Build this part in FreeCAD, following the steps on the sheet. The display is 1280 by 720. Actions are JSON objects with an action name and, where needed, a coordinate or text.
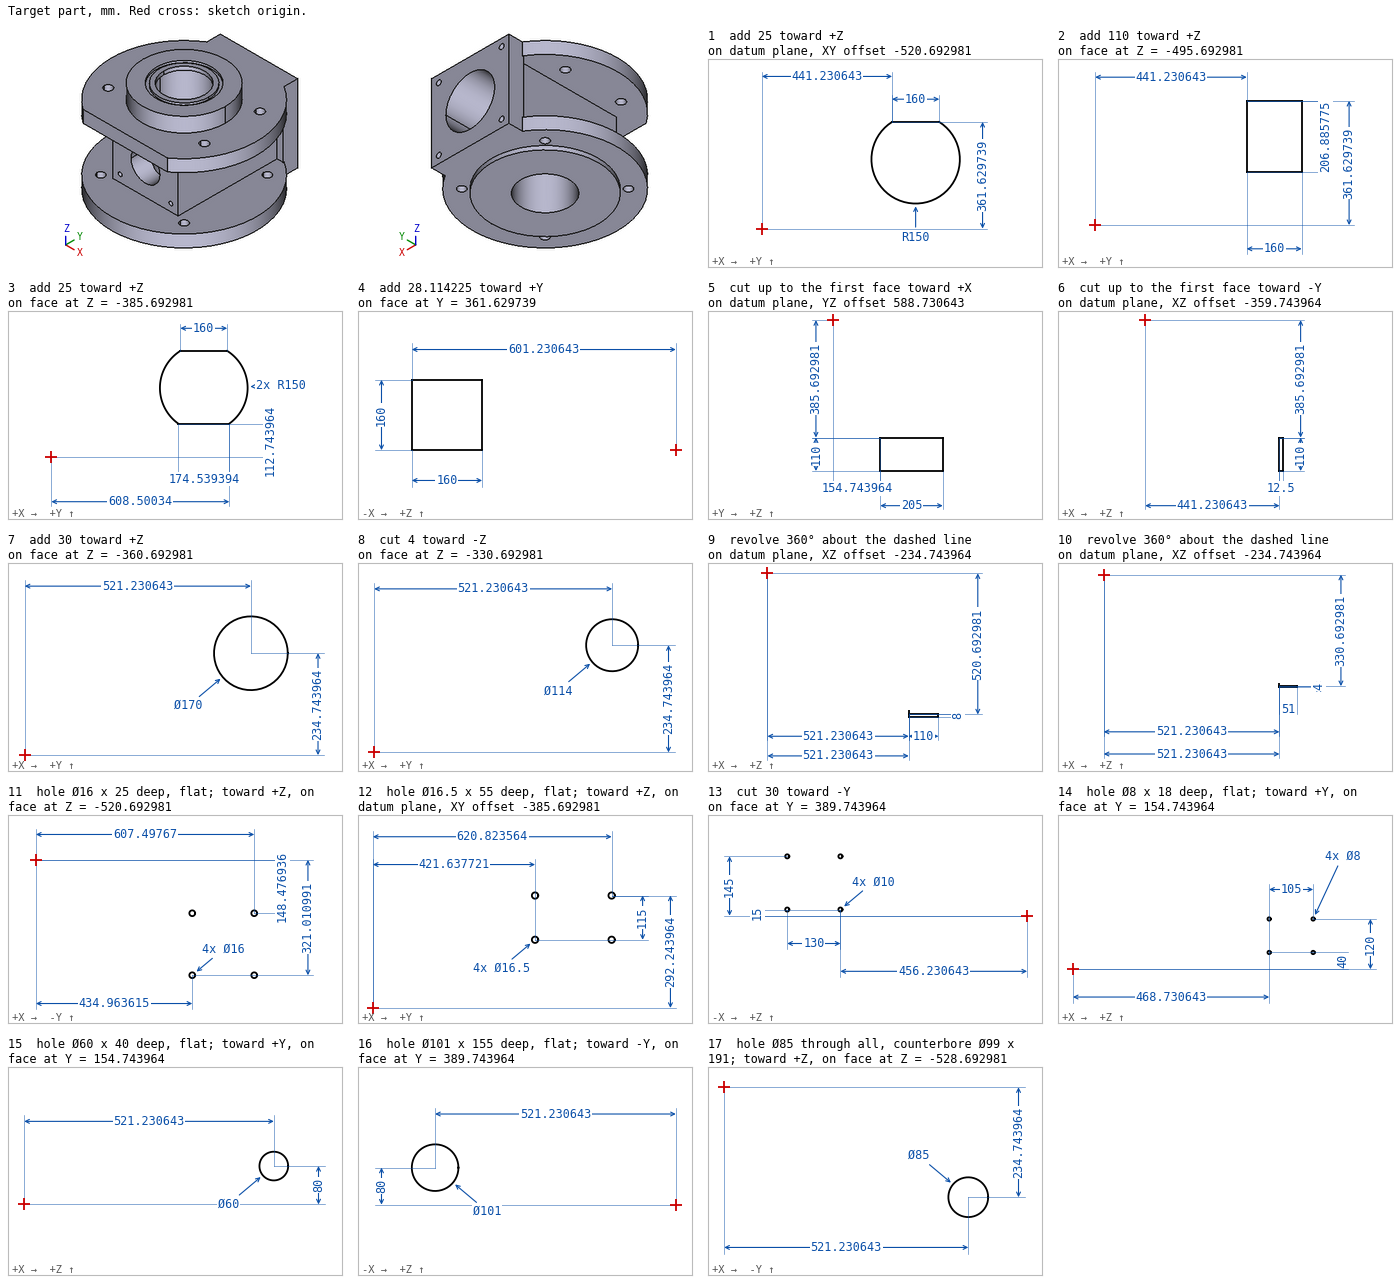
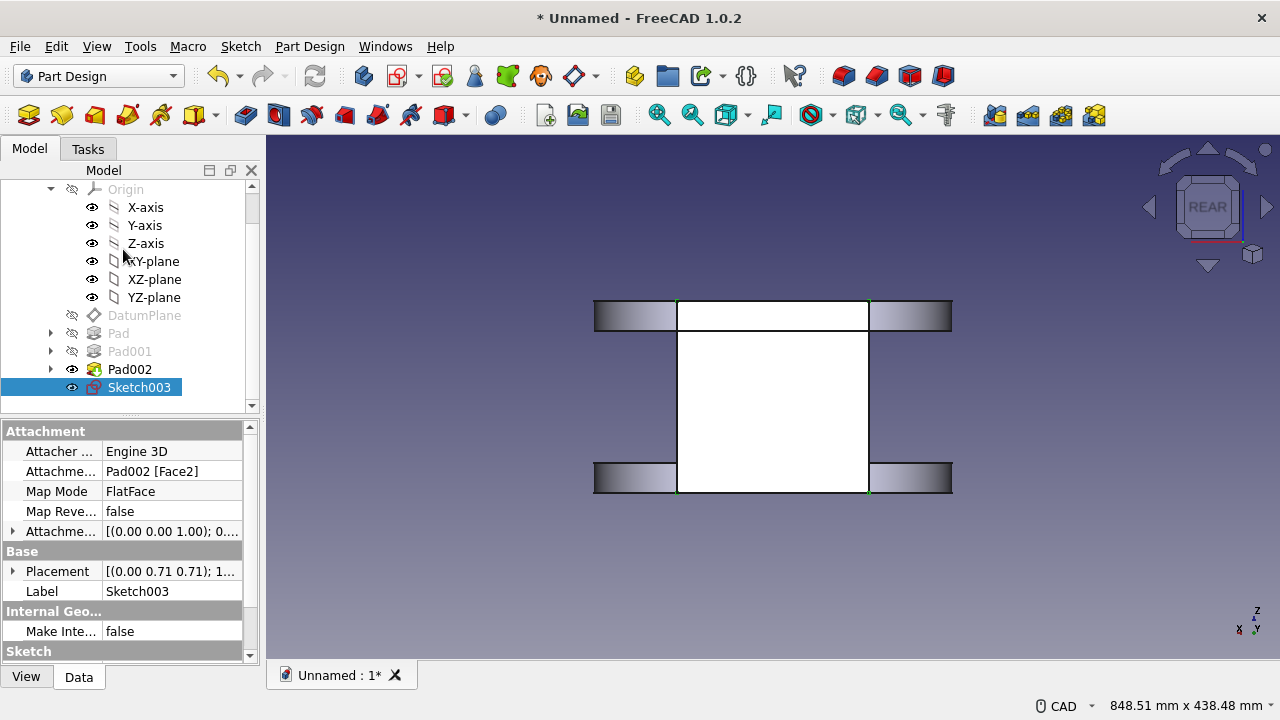
{"action": "left_click", "coordinate": [29, 116]}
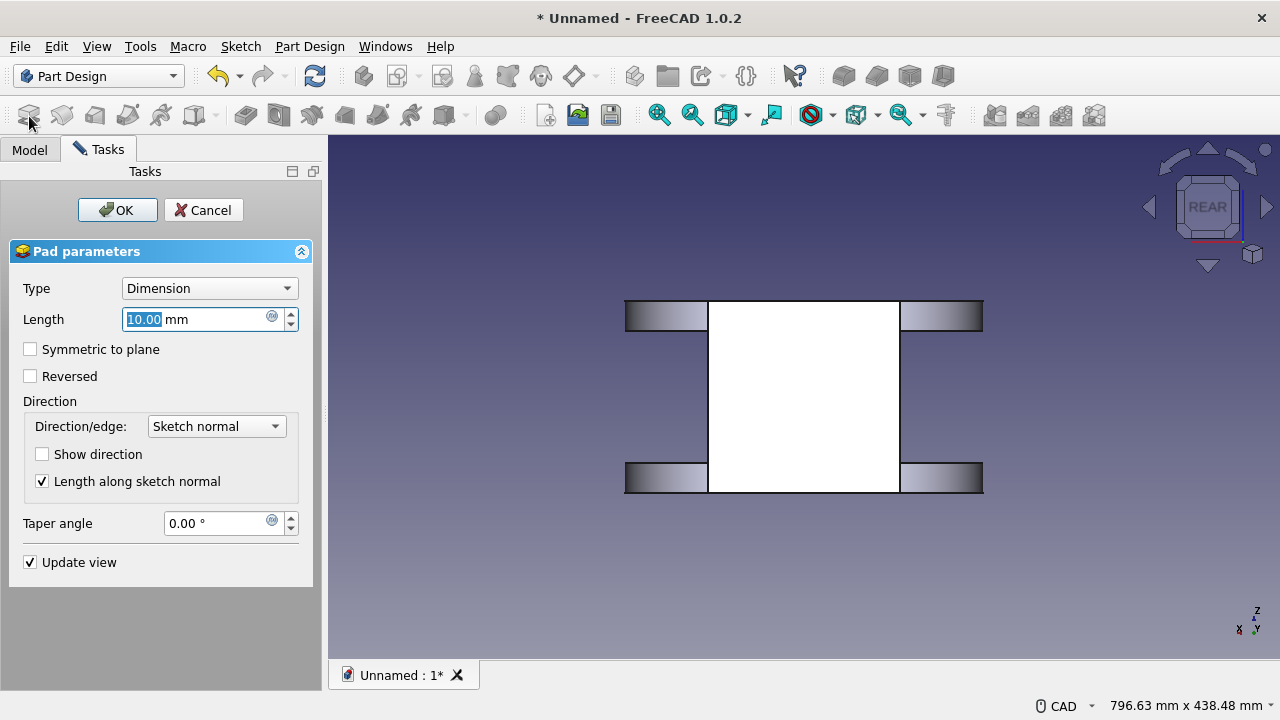
{"action": "type", "text": "28.114225"}
{"action": "key", "text": "Tab"}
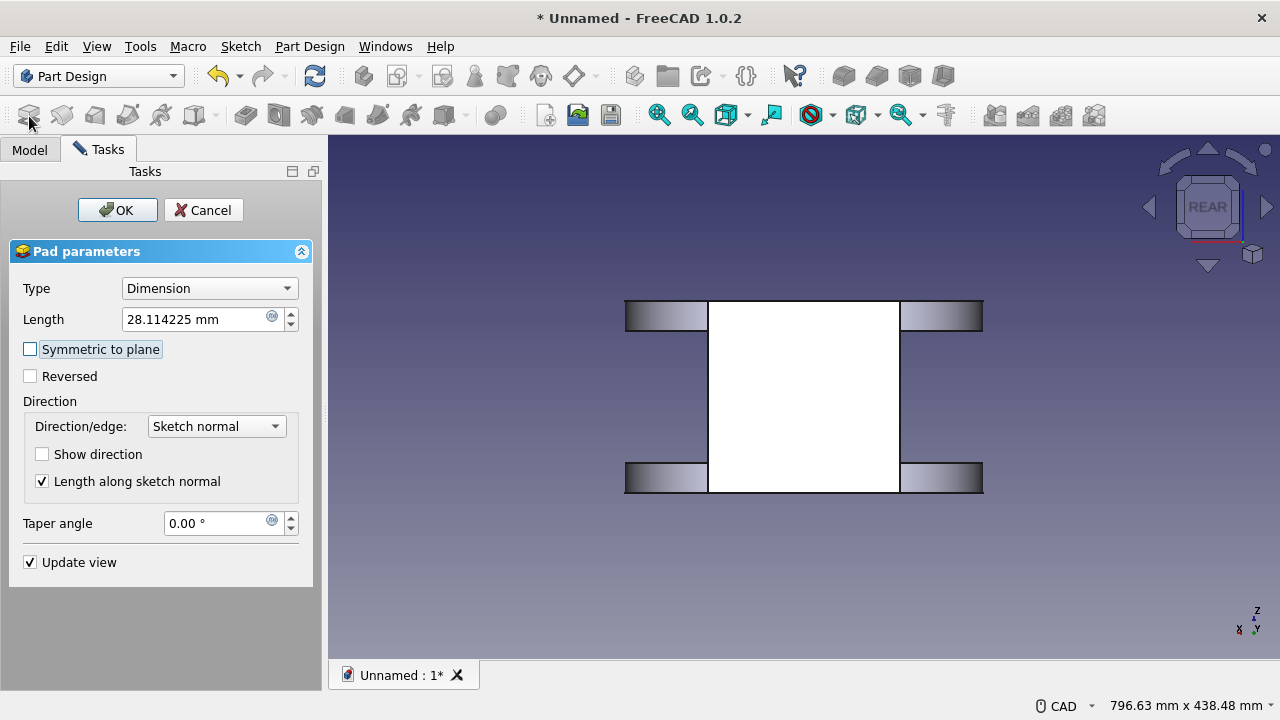
{"action": "left_click", "coordinate": [118, 210]}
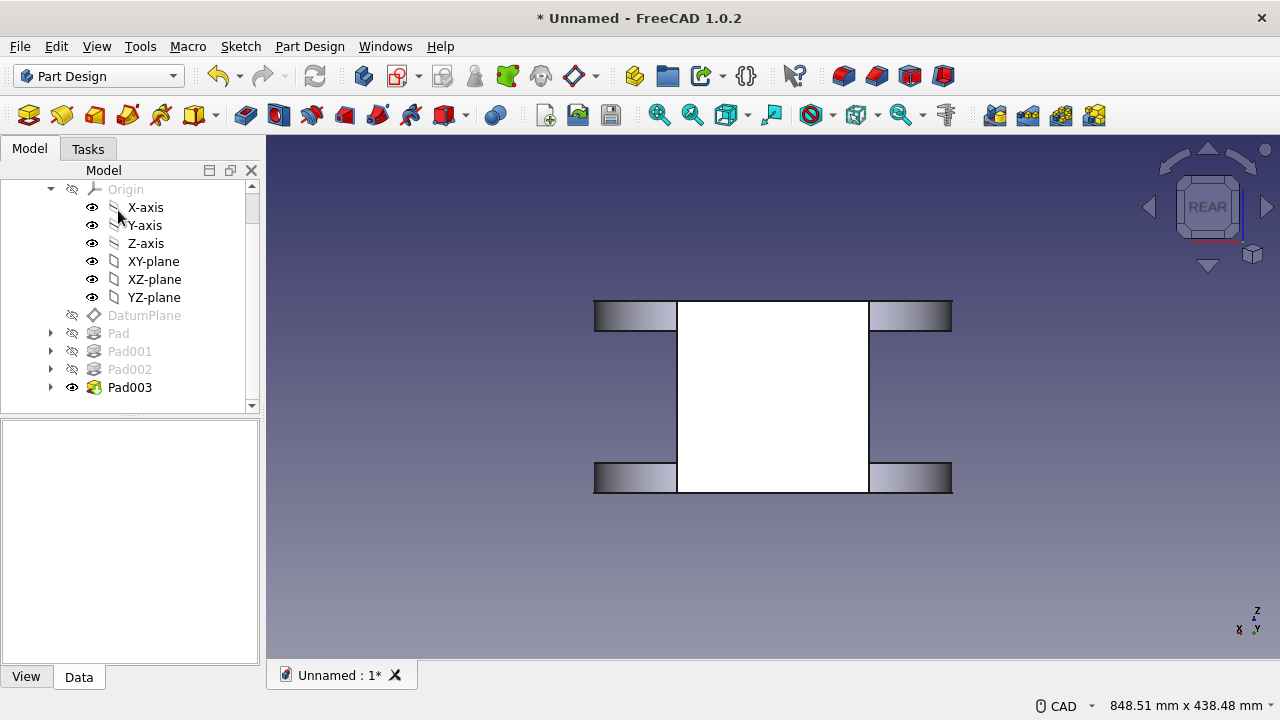
{"action": "left_click", "coordinate": [660, 116]}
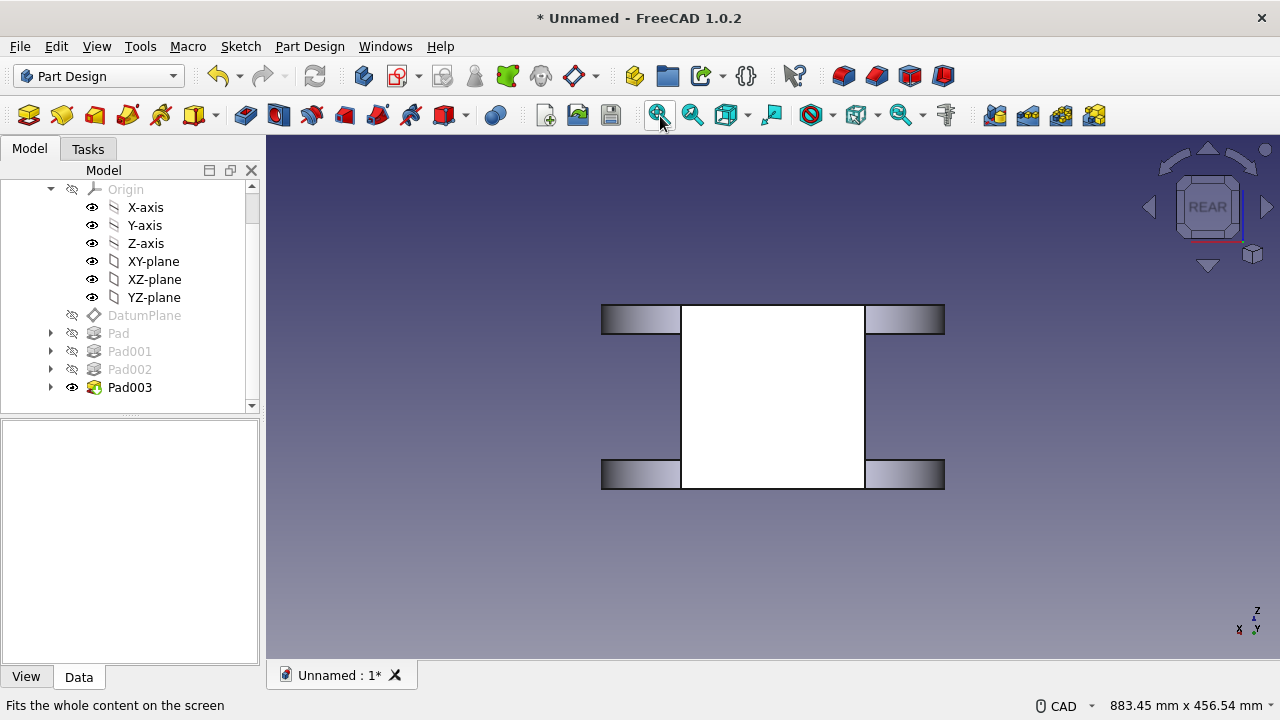
{"action": "left_click", "coordinate": [137, 297]}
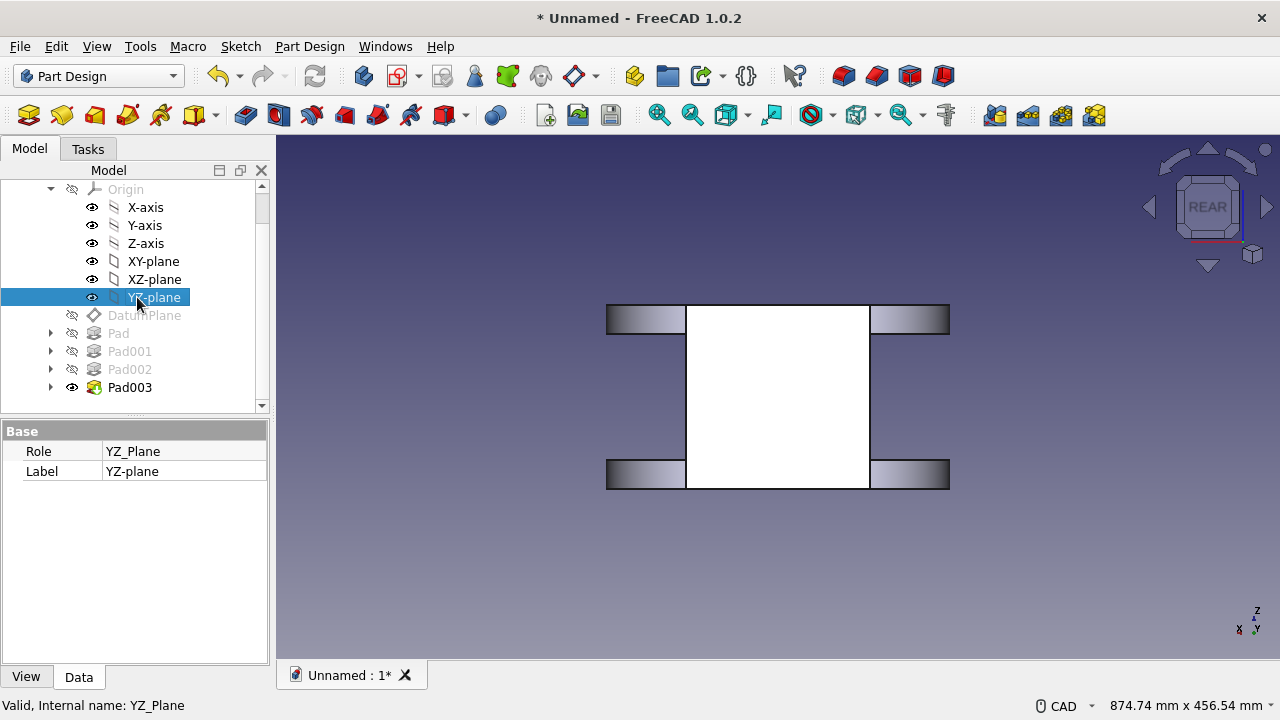
{"action": "left_click", "coordinate": [574, 76]}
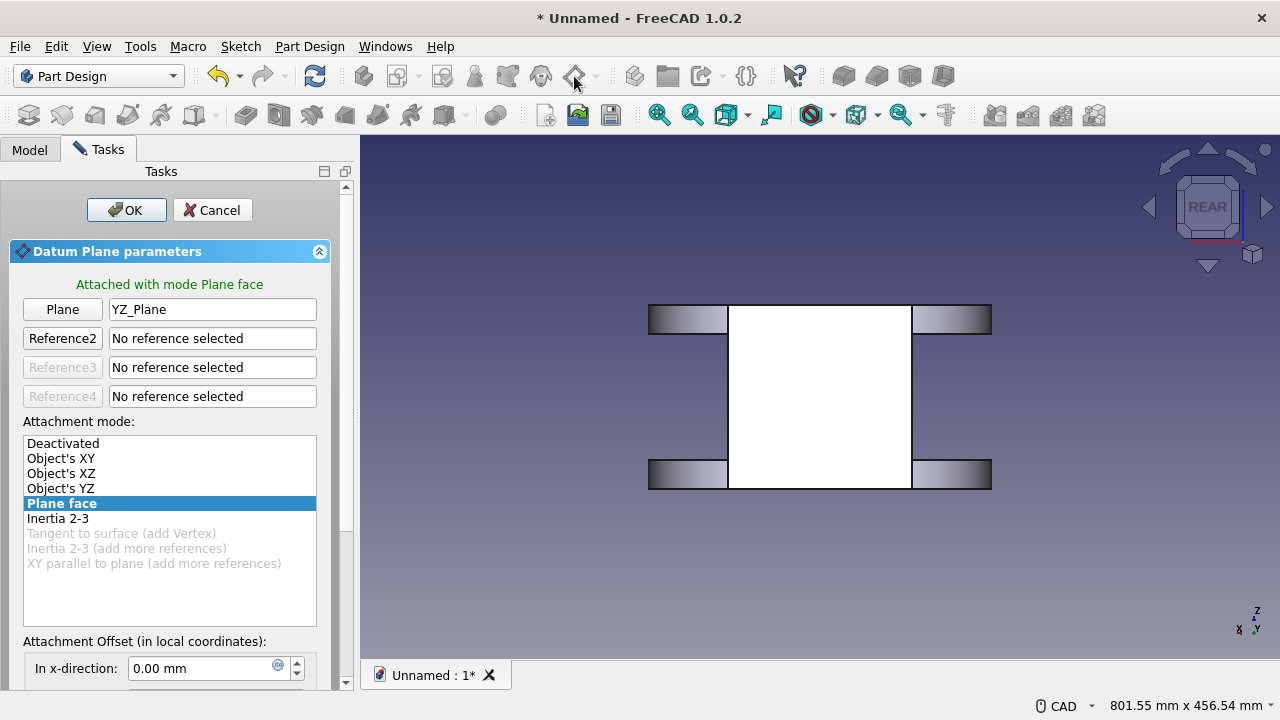
{"action": "scroll", "coordinate": [346, 436], "scroll_direction": "down", "scroll_amount": 2}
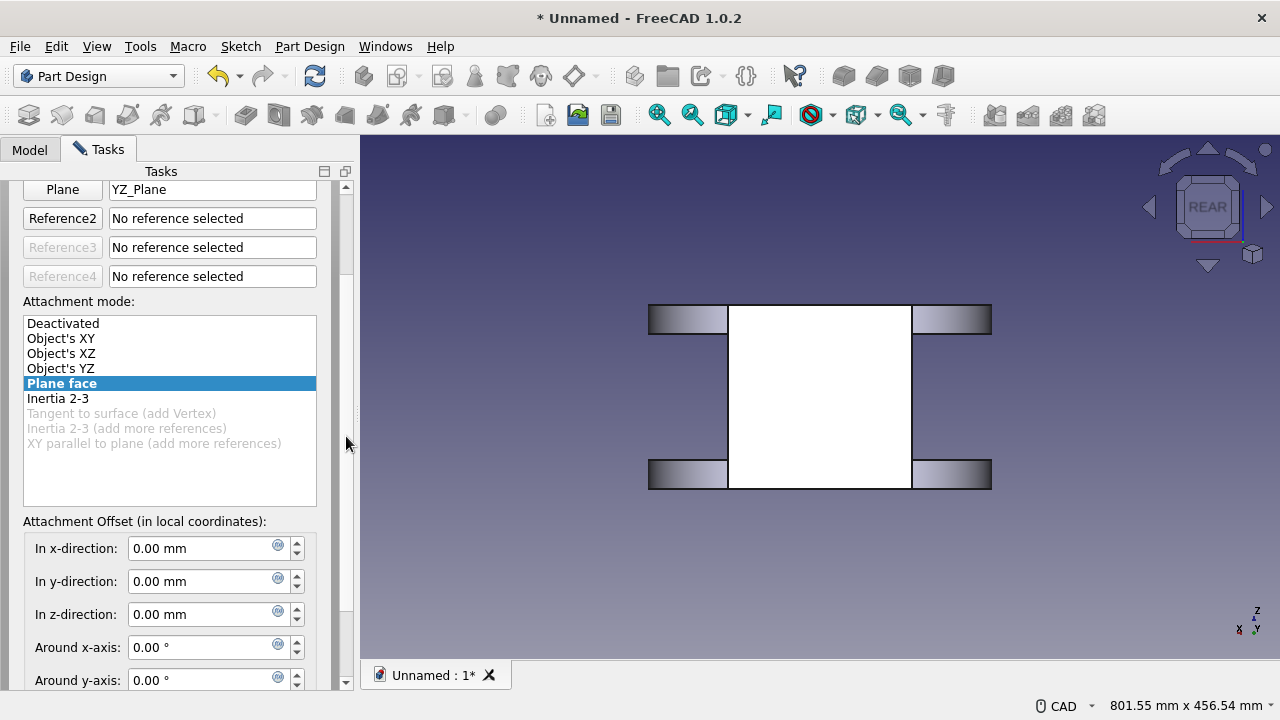
{"action": "triple_click", "coordinate": [210, 614]}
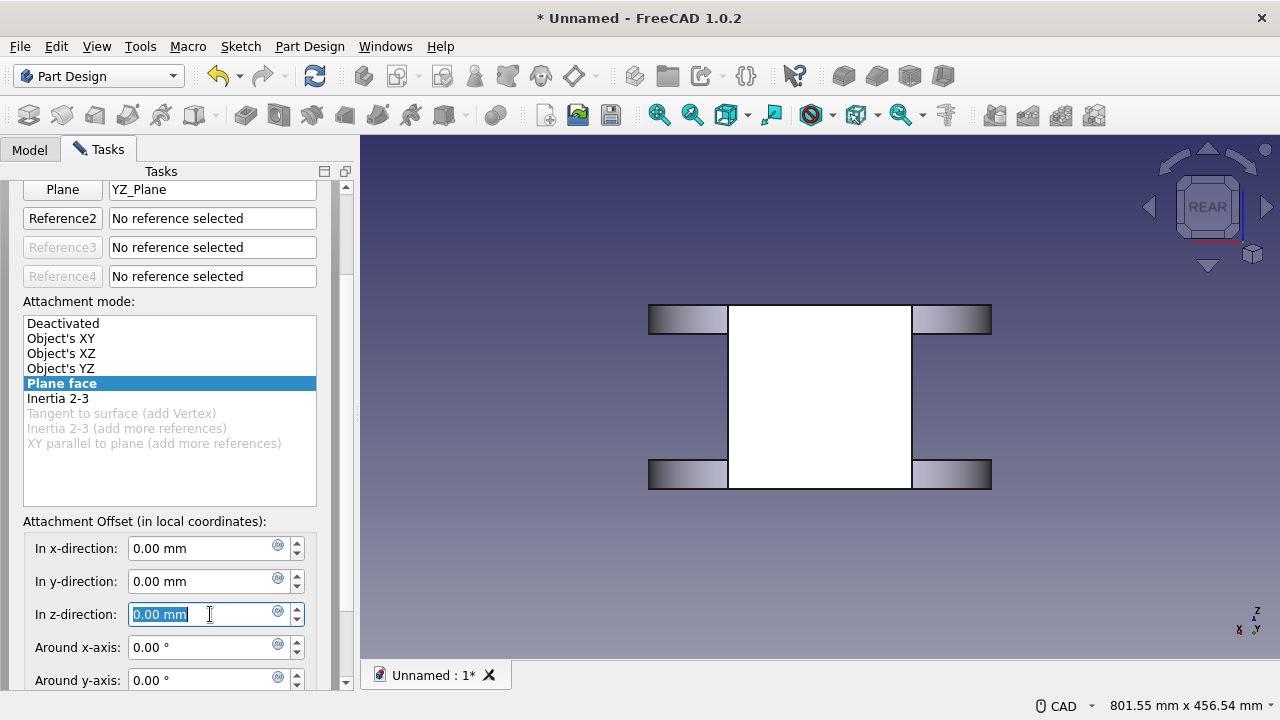
{"action": "type", "text": "588.730643"}
{"action": "key", "text": "Tab"}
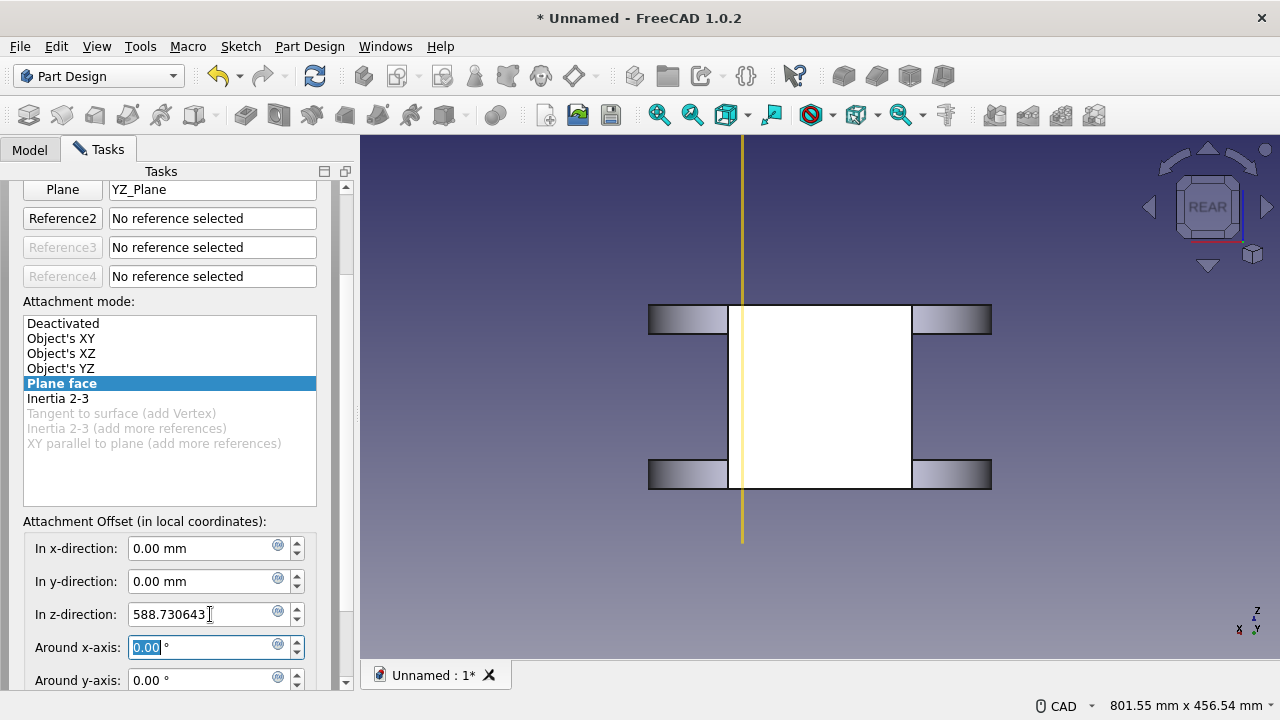
{"action": "scroll", "coordinate": [346, 436], "scroll_direction": "up", "scroll_amount": 3}